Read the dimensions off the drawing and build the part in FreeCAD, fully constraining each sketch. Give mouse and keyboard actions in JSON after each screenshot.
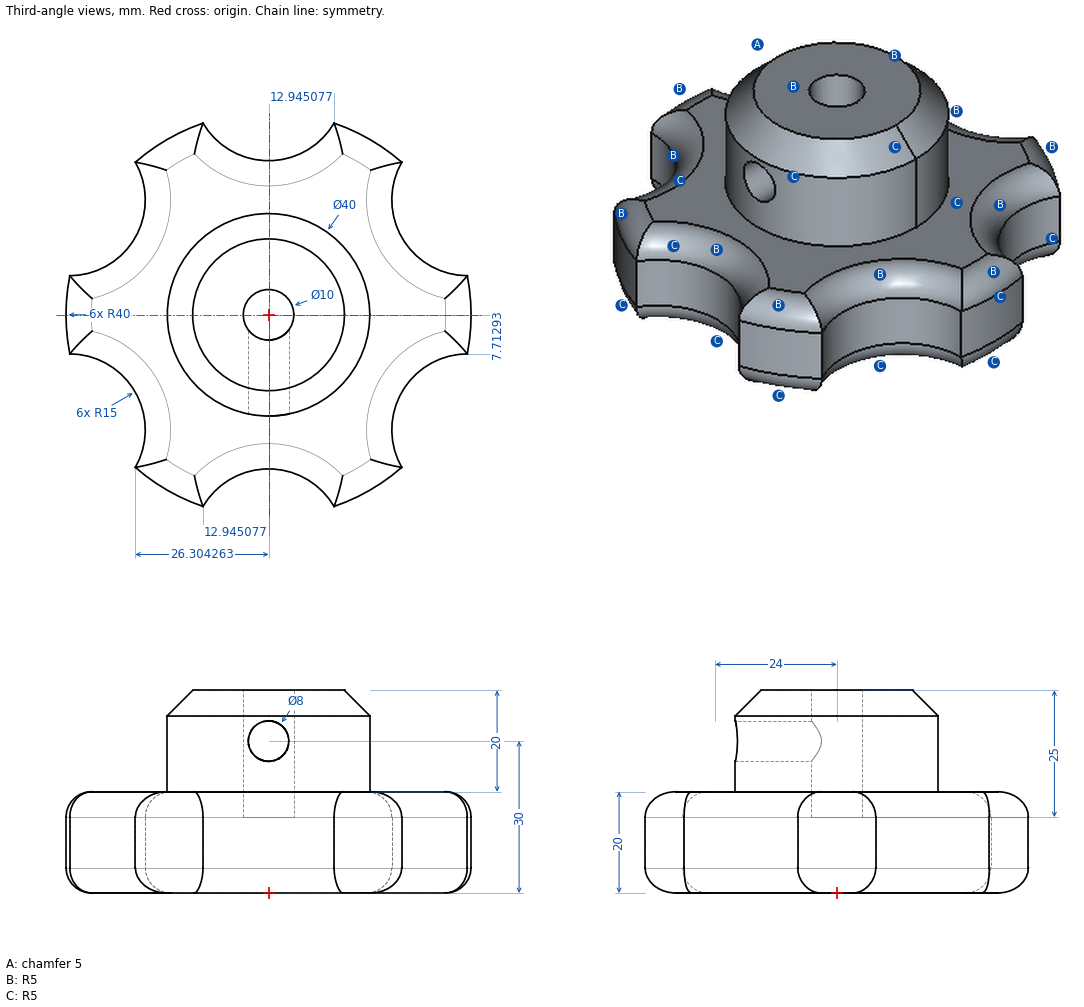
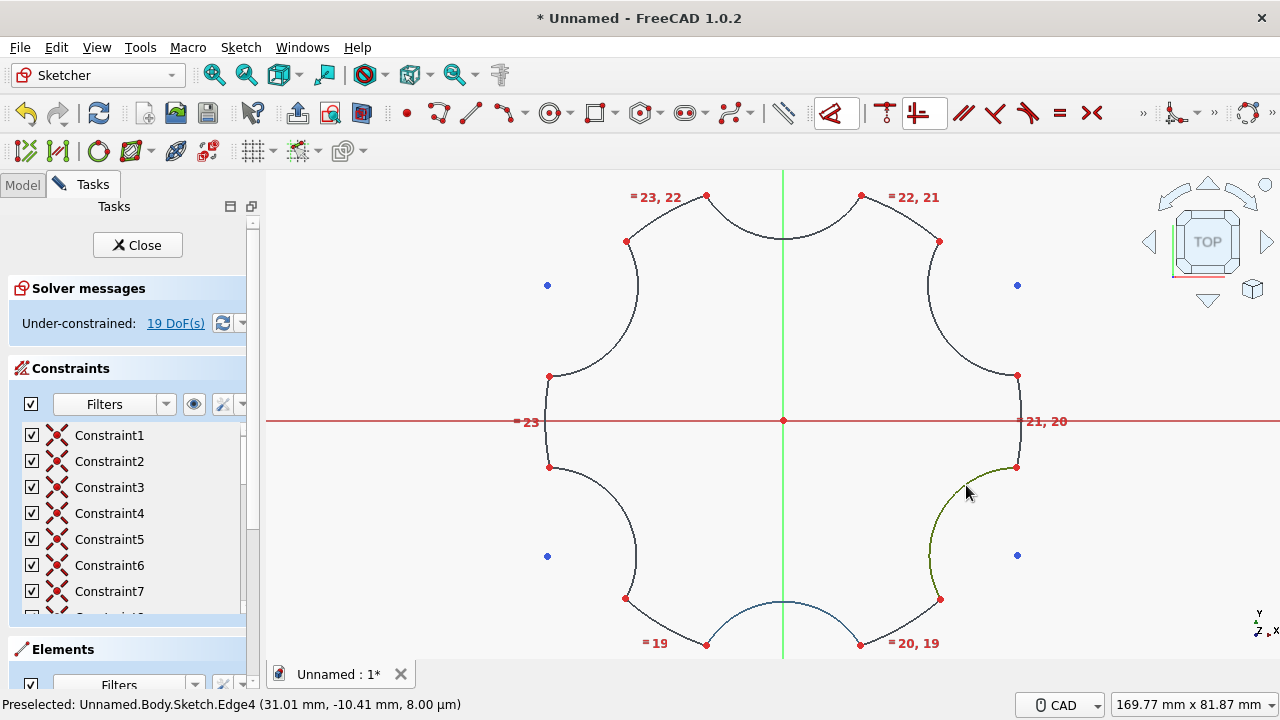
{"action": "left_click", "coordinate": [928, 295]}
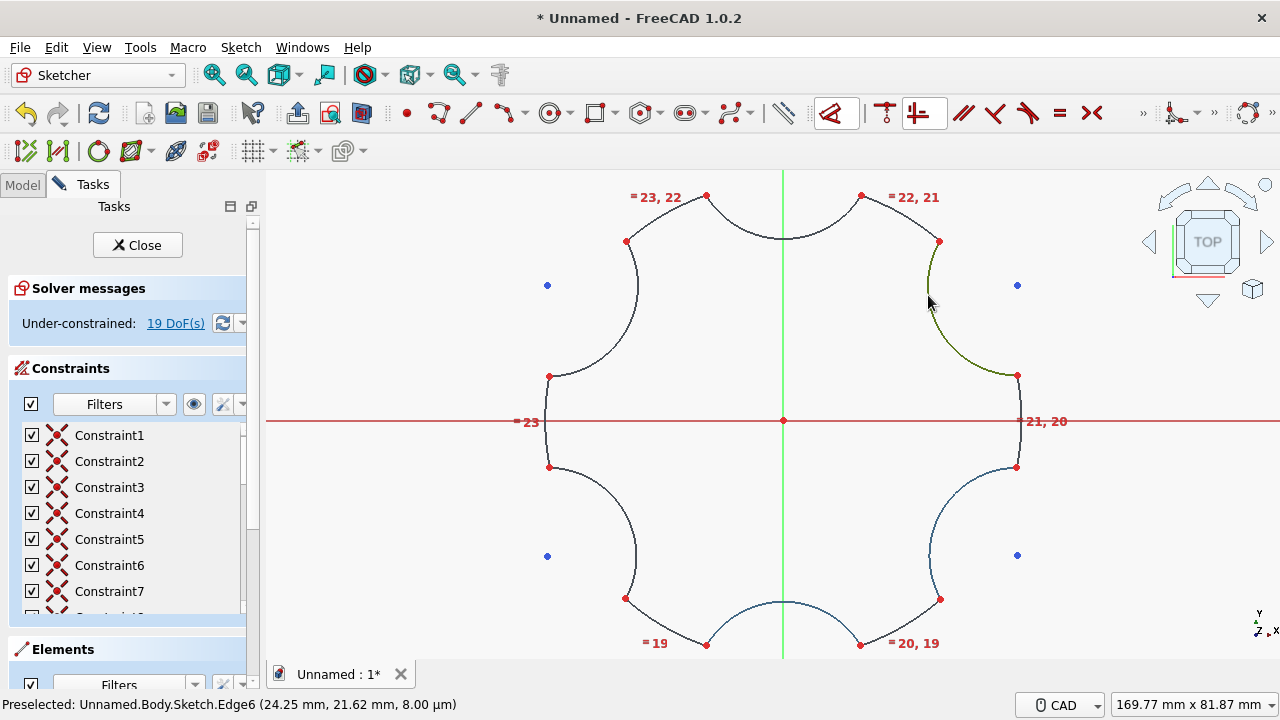
{"action": "left_click", "coordinate": [747, 231]}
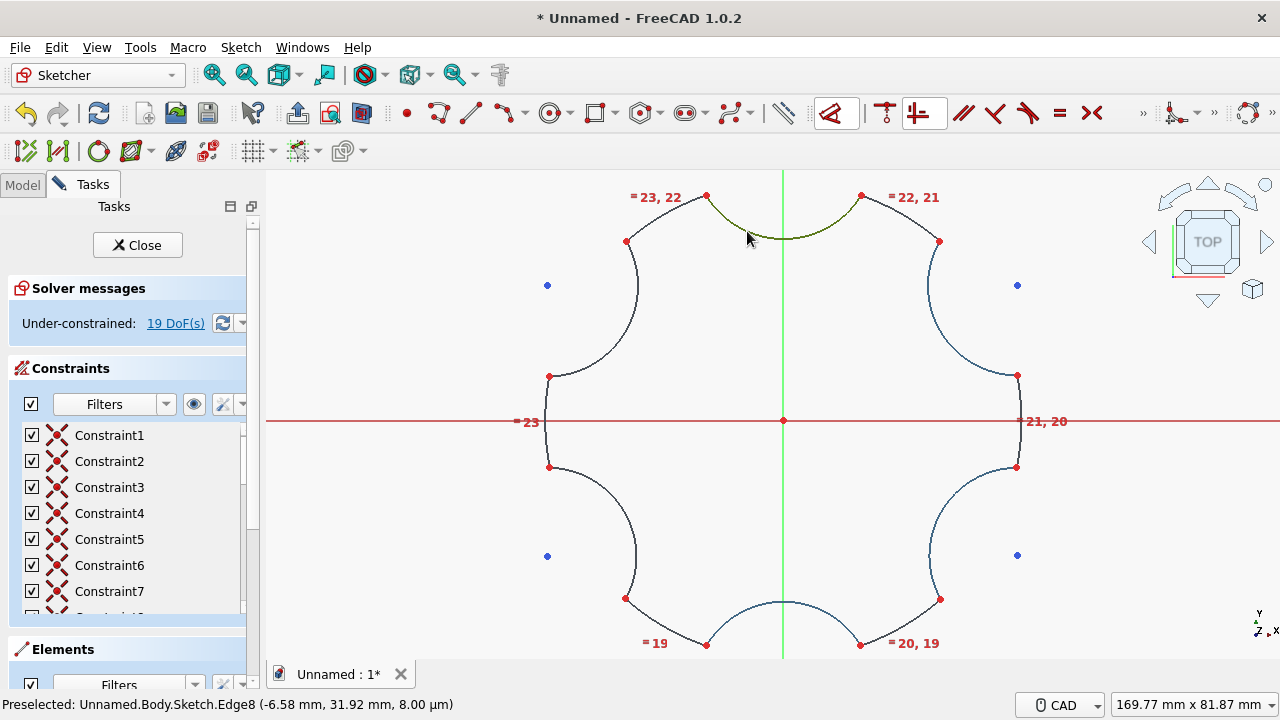
{"action": "left_click", "coordinate": [601, 359]}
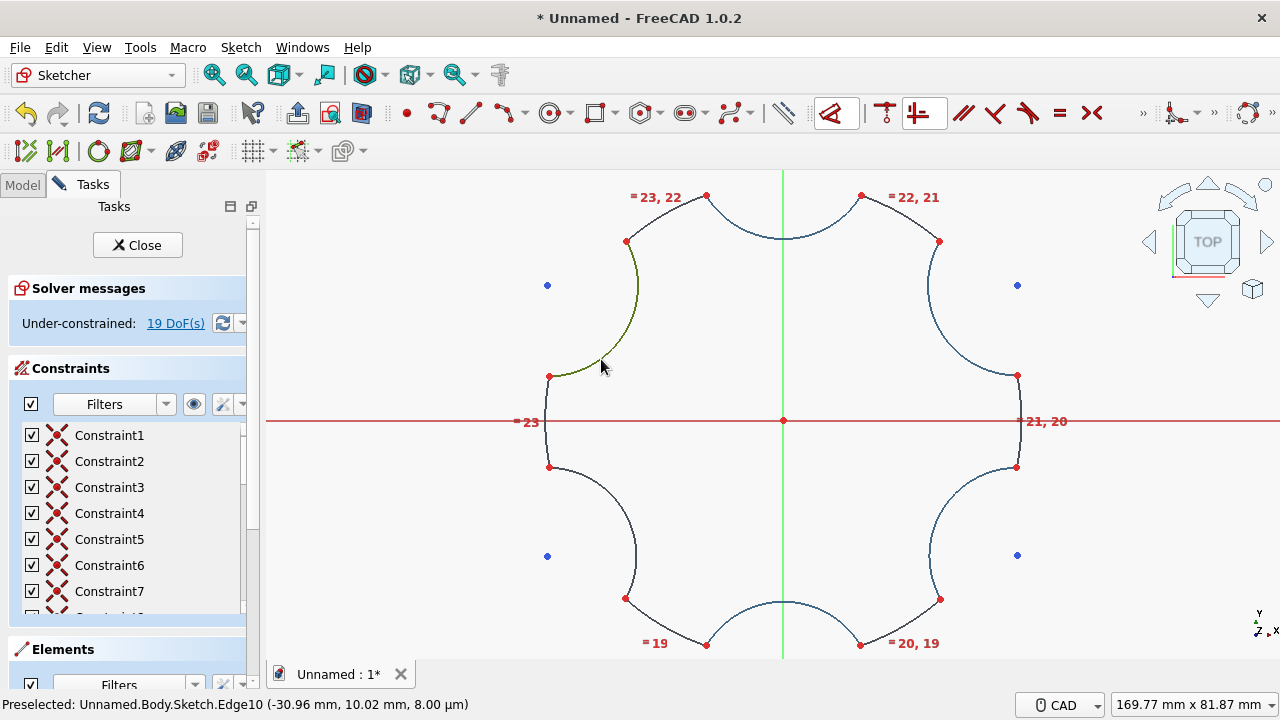
{"action": "left_click", "coordinate": [636, 546]}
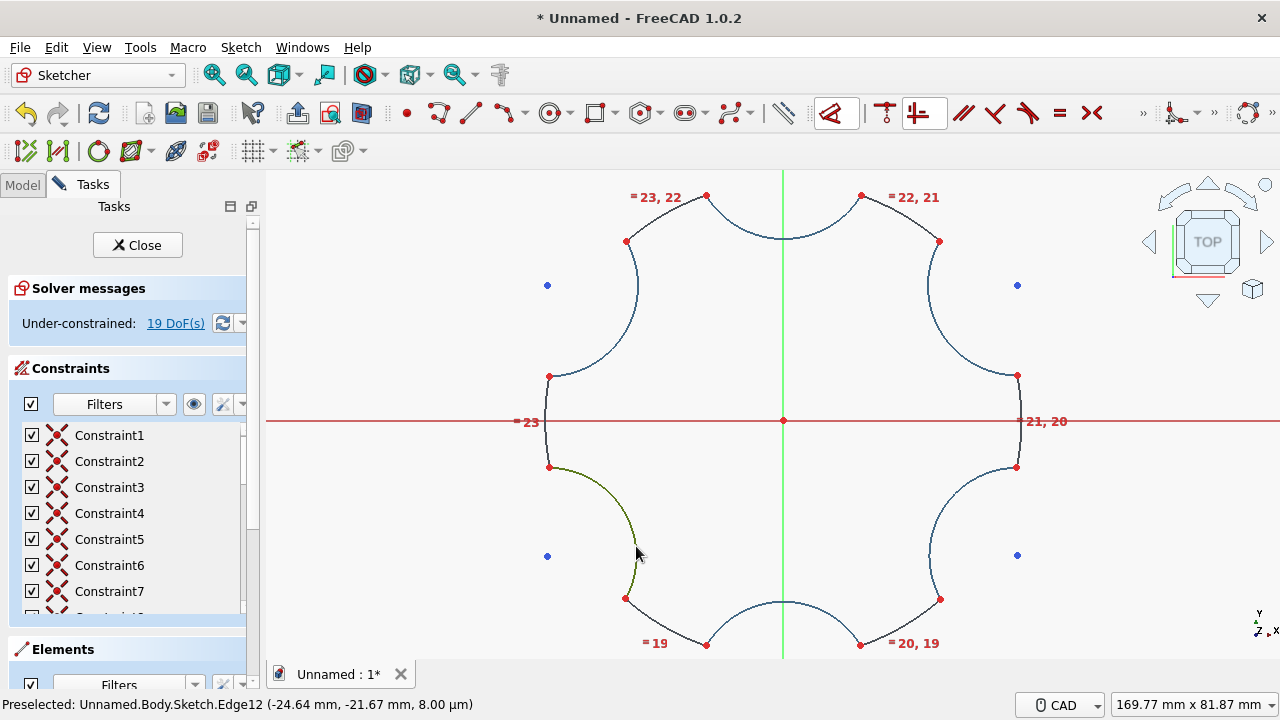
{"action": "left_click", "coordinate": [1060, 114]}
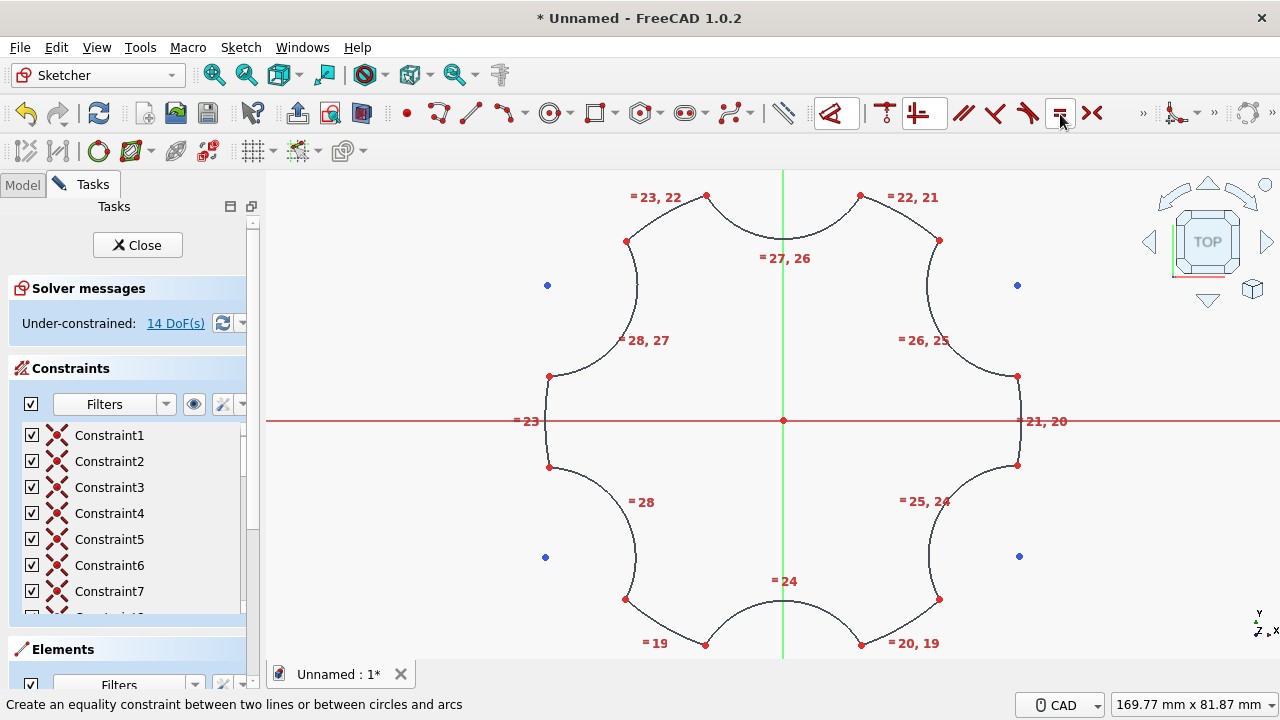
{"action": "scroll", "coordinate": [544, 402], "scroll_direction": "down", "scroll_amount": 2}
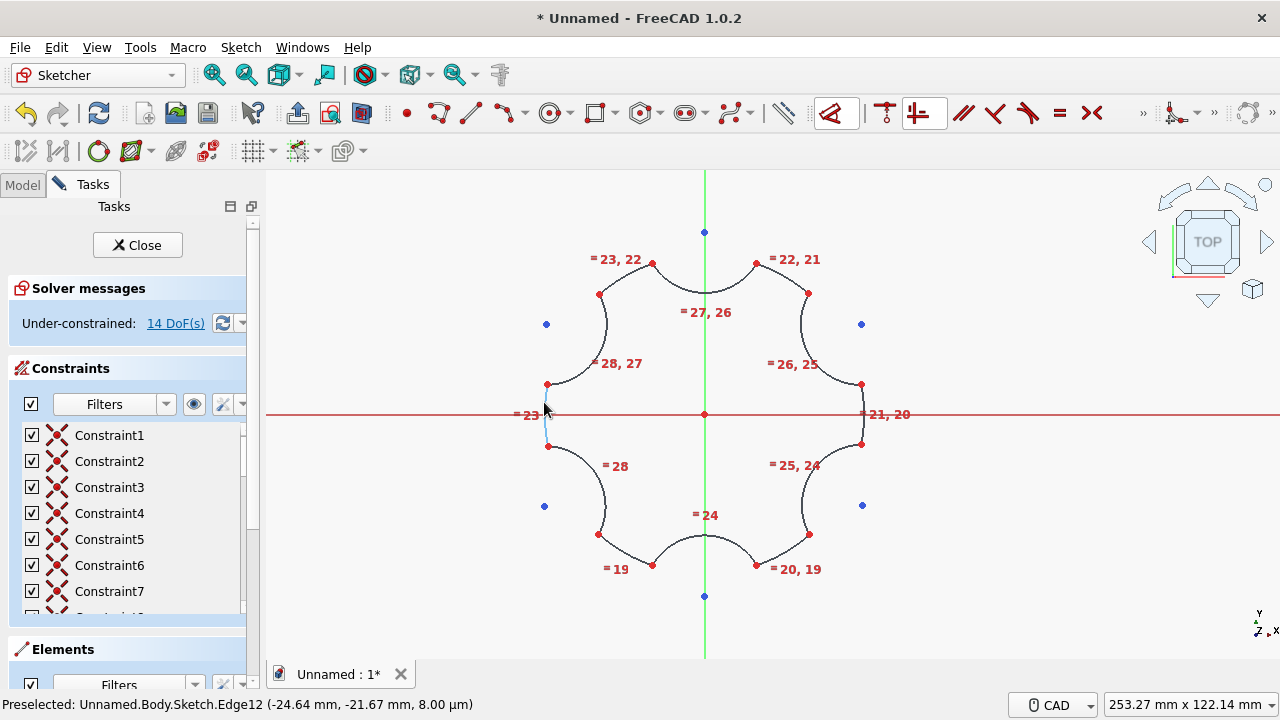
{"action": "left_click", "coordinate": [705, 596]}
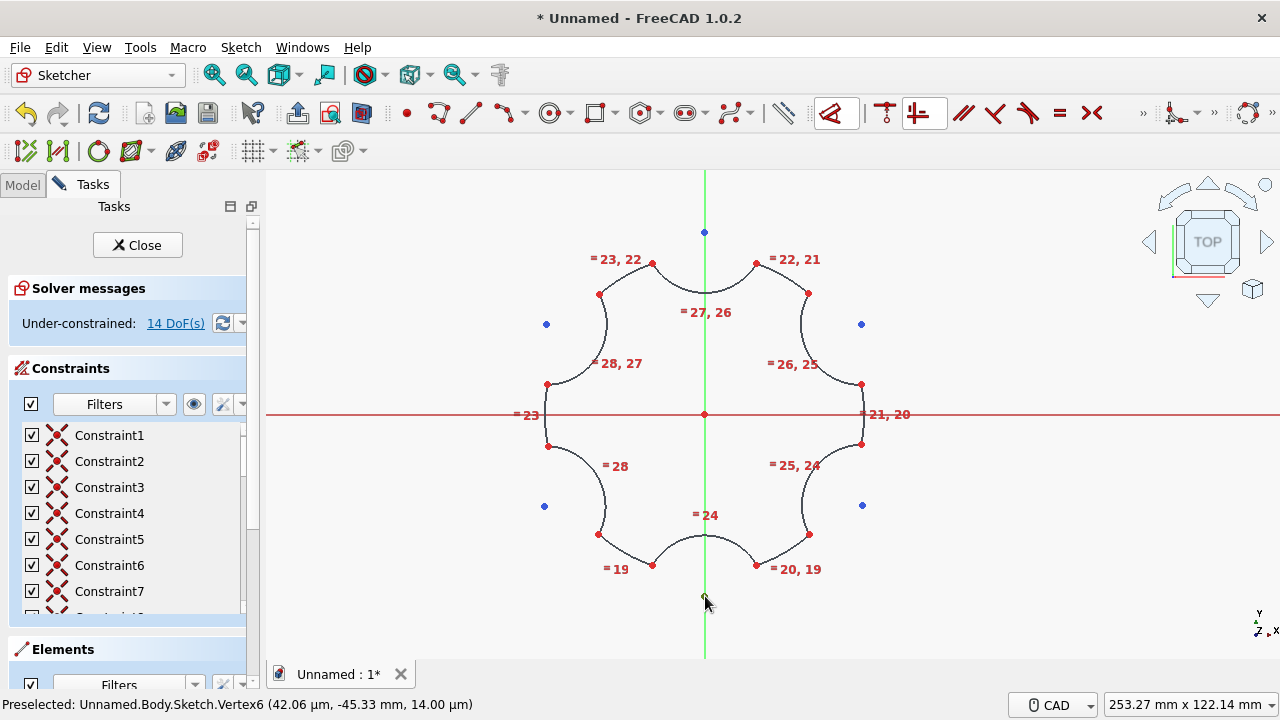
{"action": "left_click", "coordinate": [705, 569]}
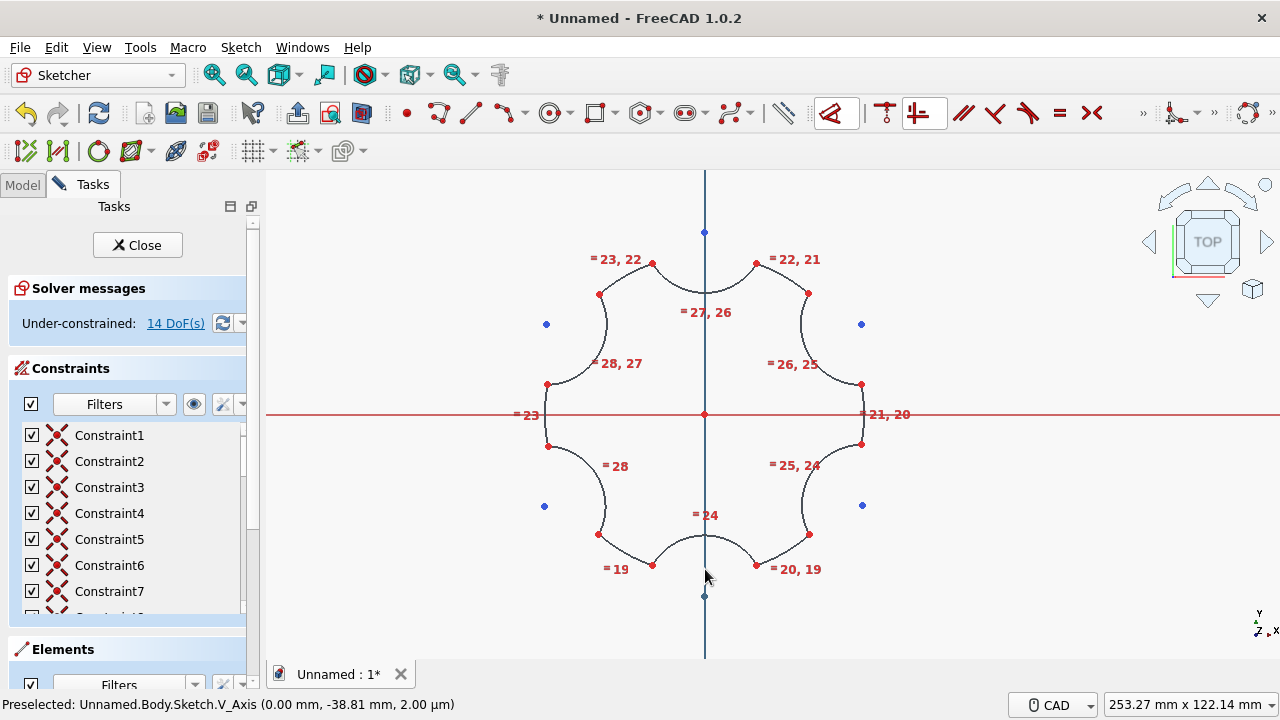
{"action": "left_click", "coordinate": [886, 114]}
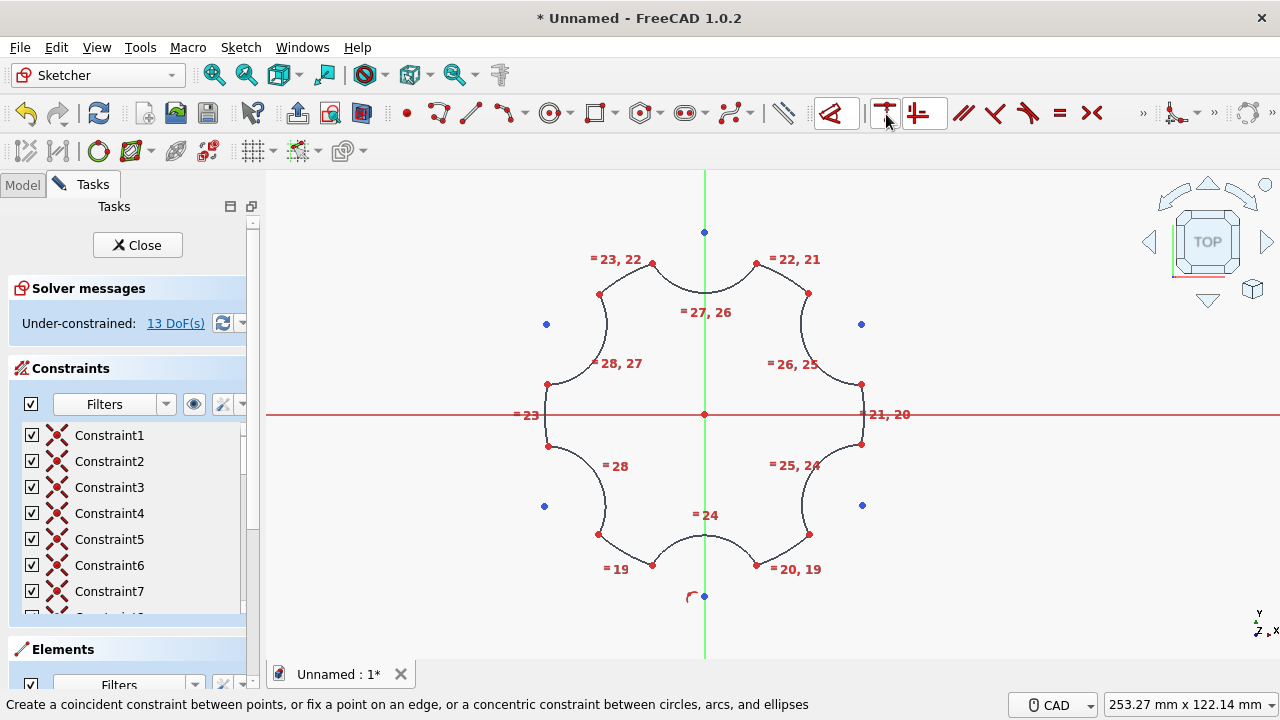
{"action": "left_click", "coordinate": [705, 232]}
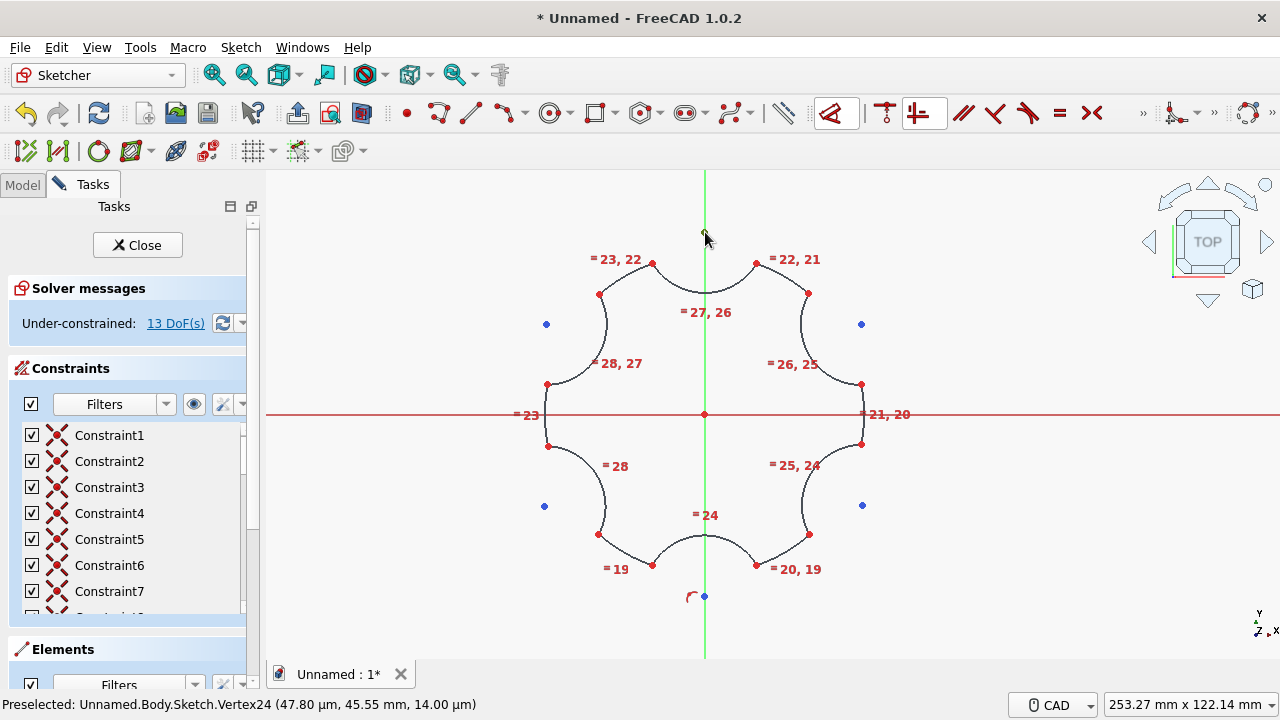
{"action": "left_click", "coordinate": [705, 569]}